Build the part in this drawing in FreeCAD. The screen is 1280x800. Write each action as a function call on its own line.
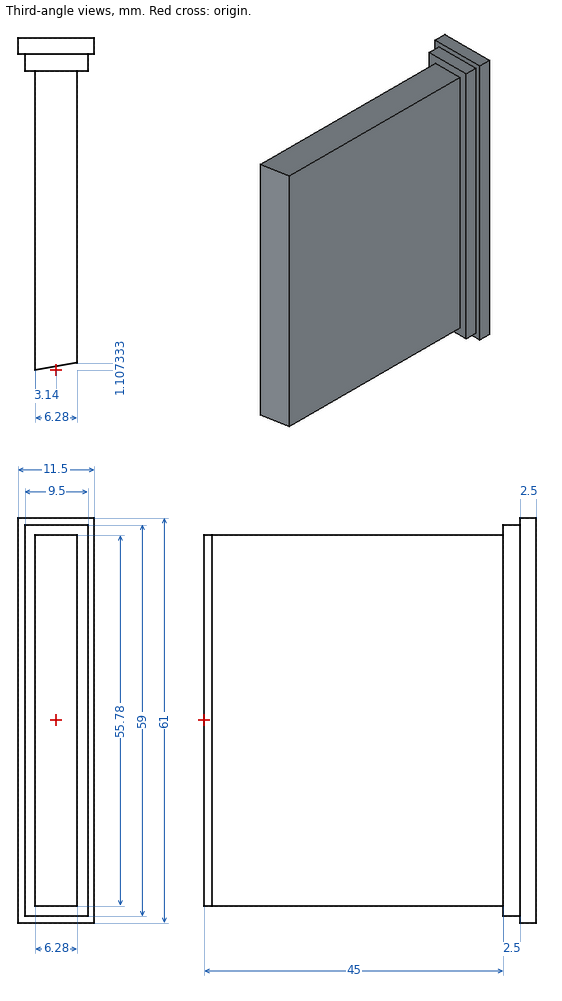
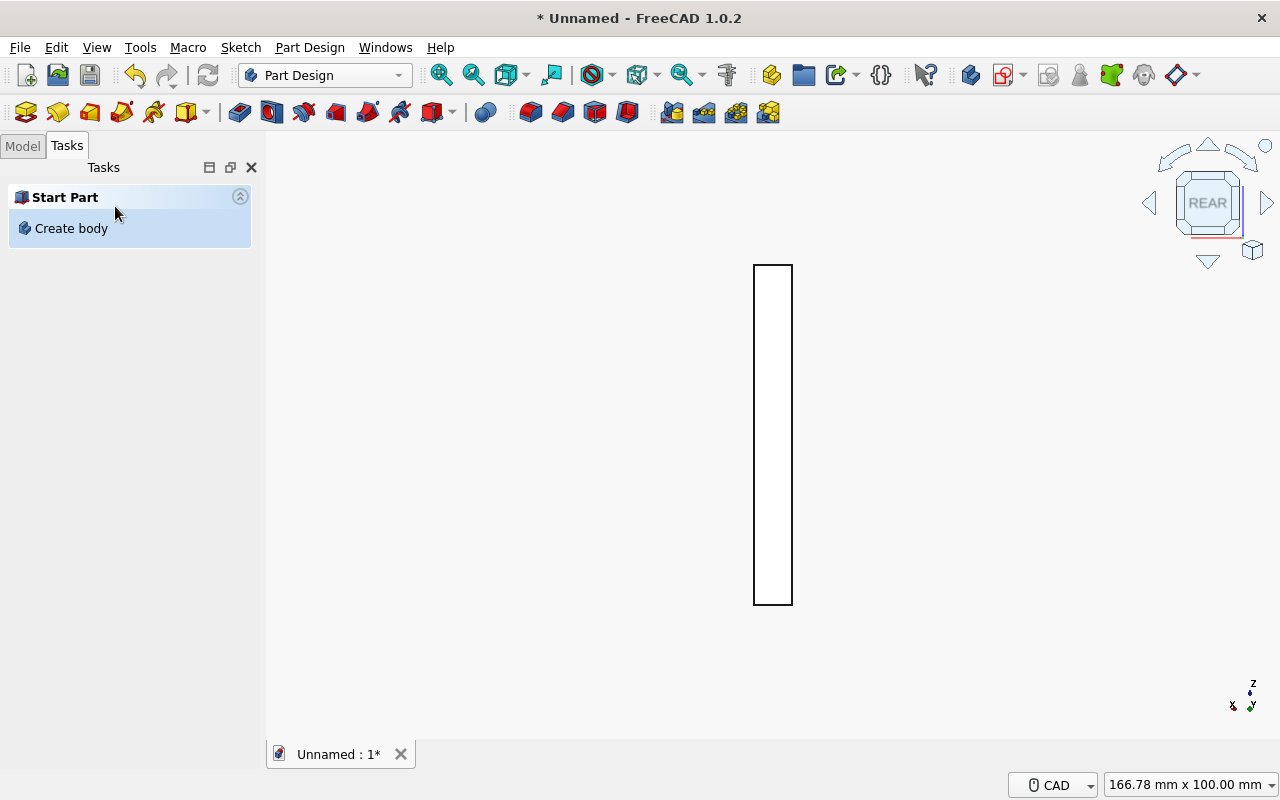
click(773, 289)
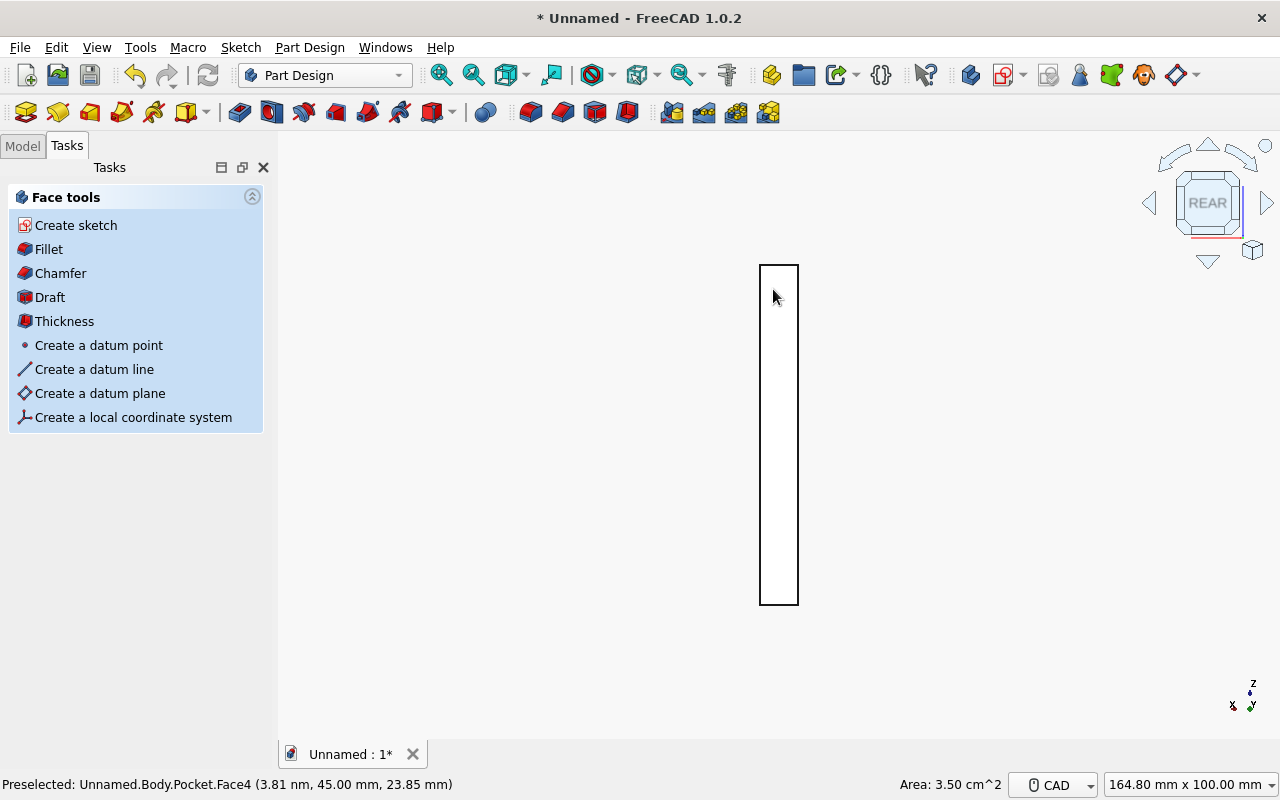
click(1004, 76)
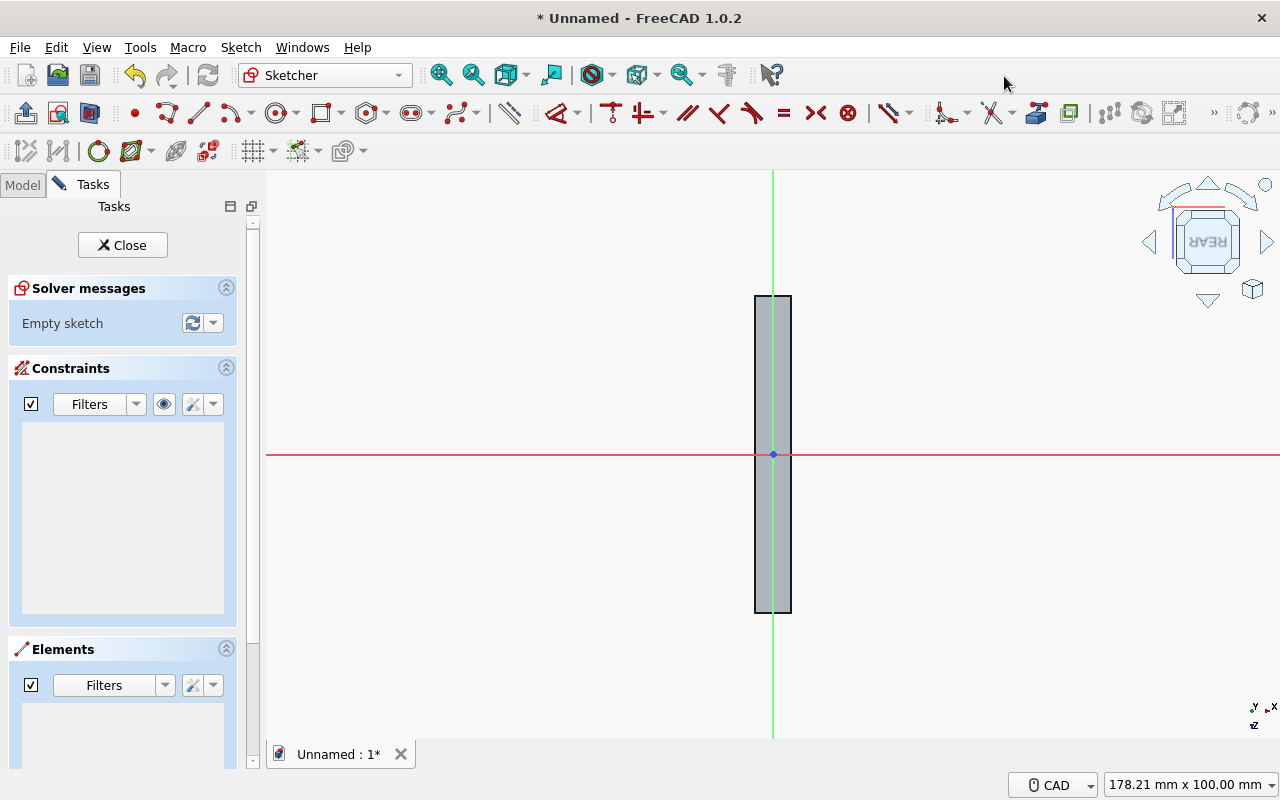
key(g)
key(v)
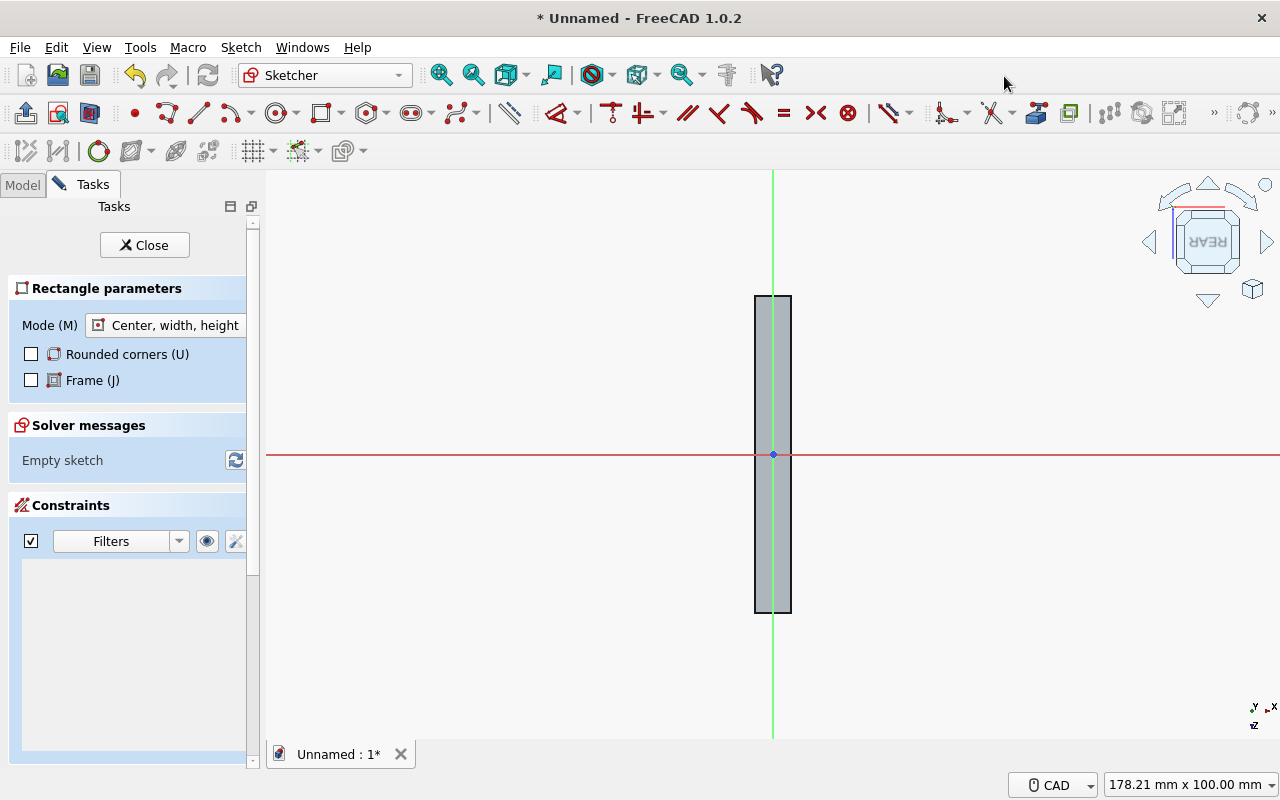
click(773, 455)
move(800, 287)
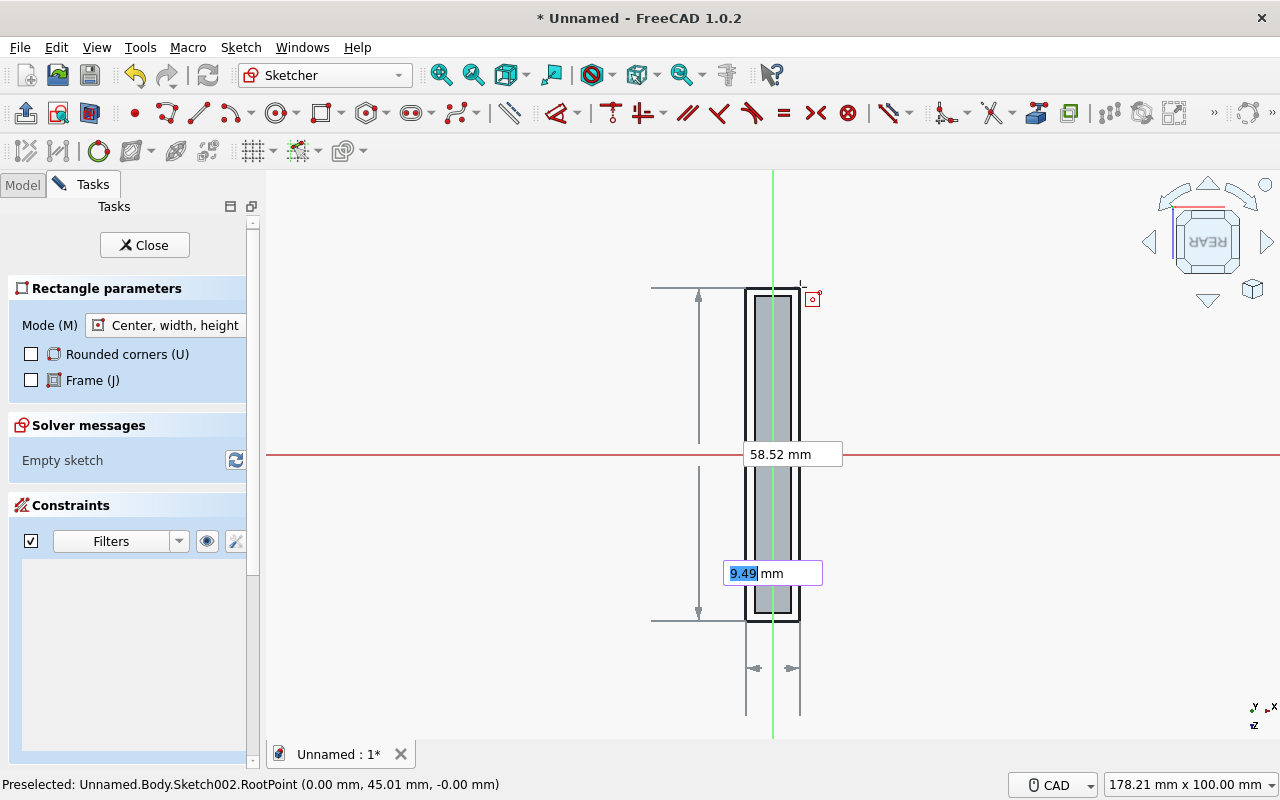
text(9.5)
key(Tab)
text(59)
key(Return)
key(Escape)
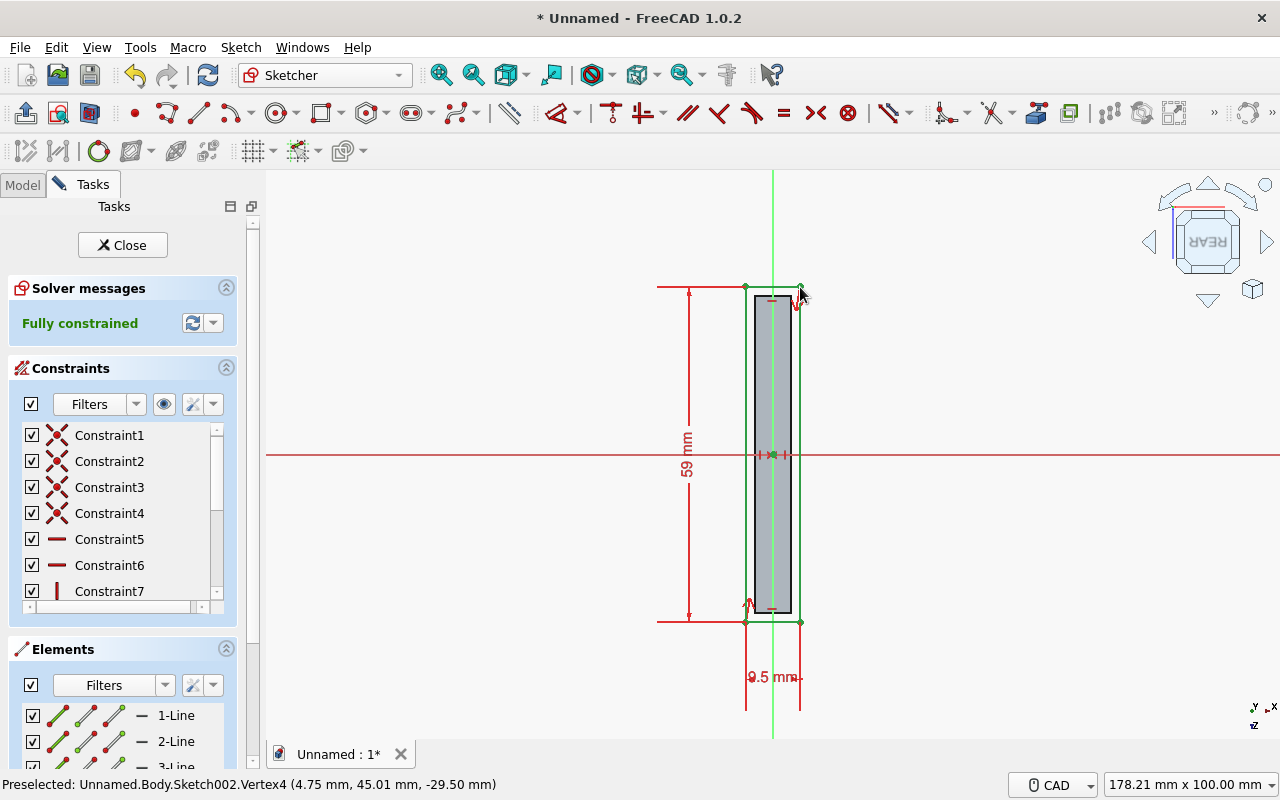
click(123, 245)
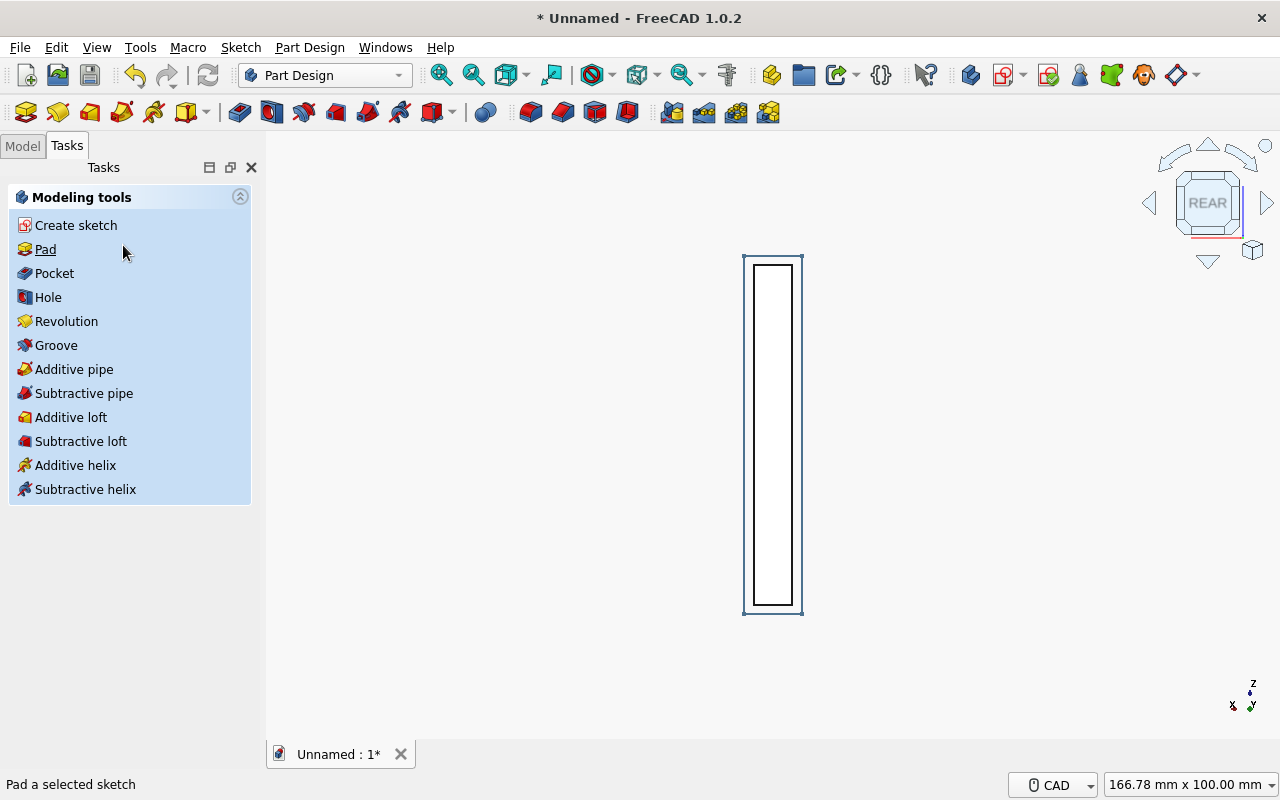
click(26, 112)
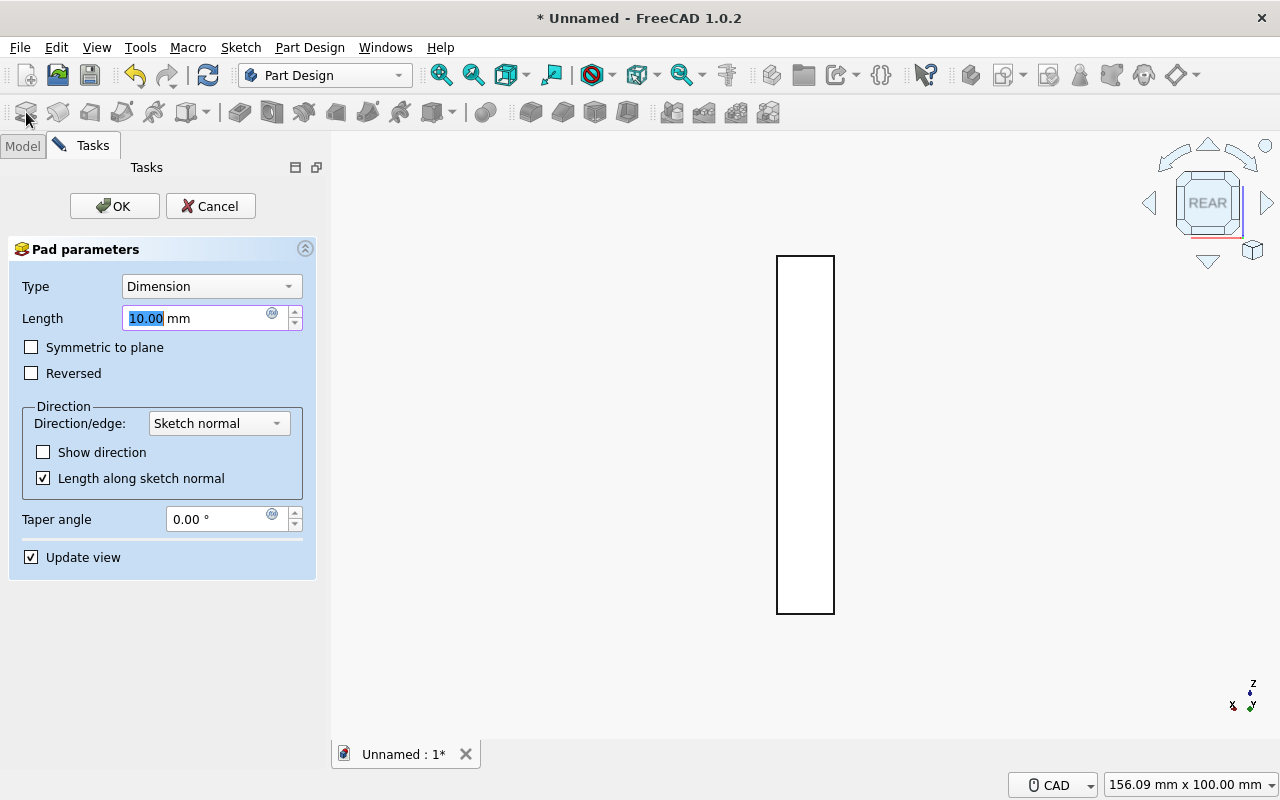
text(2.5)
key(Tab)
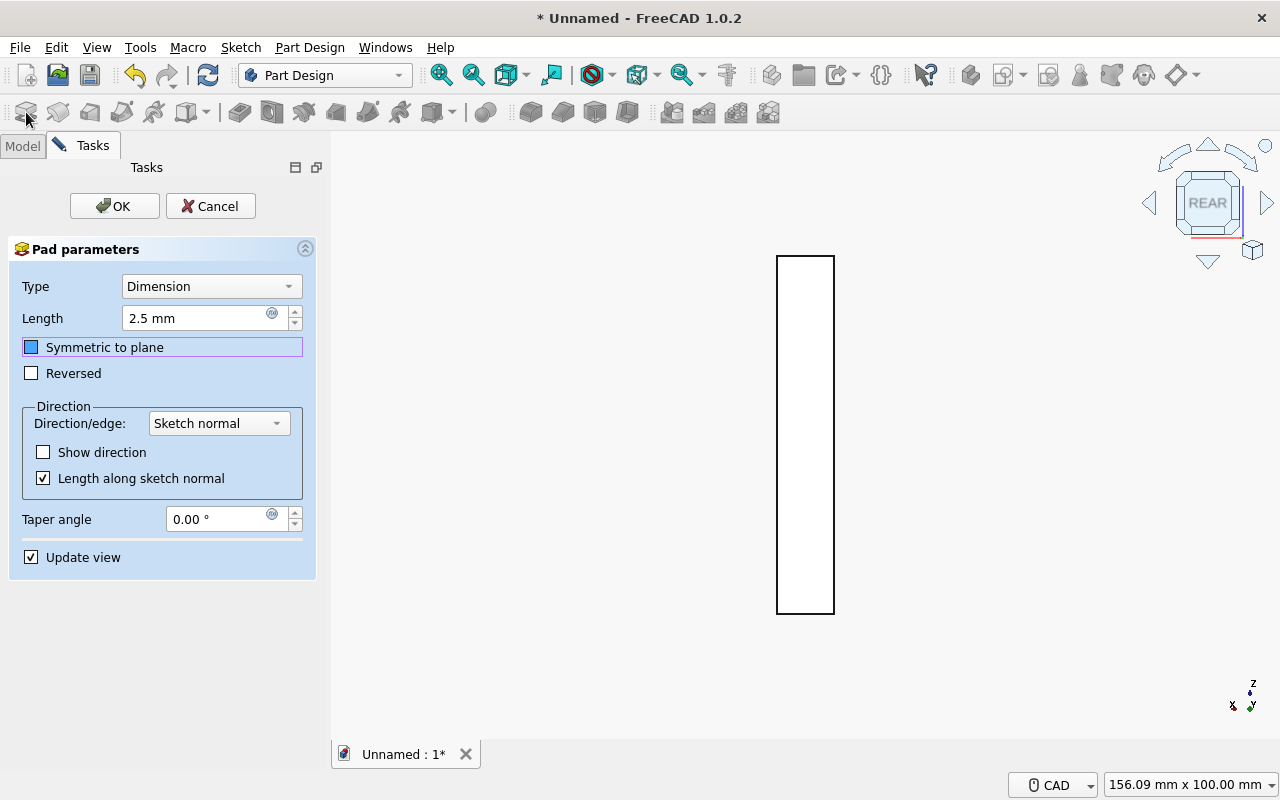
click(115, 206)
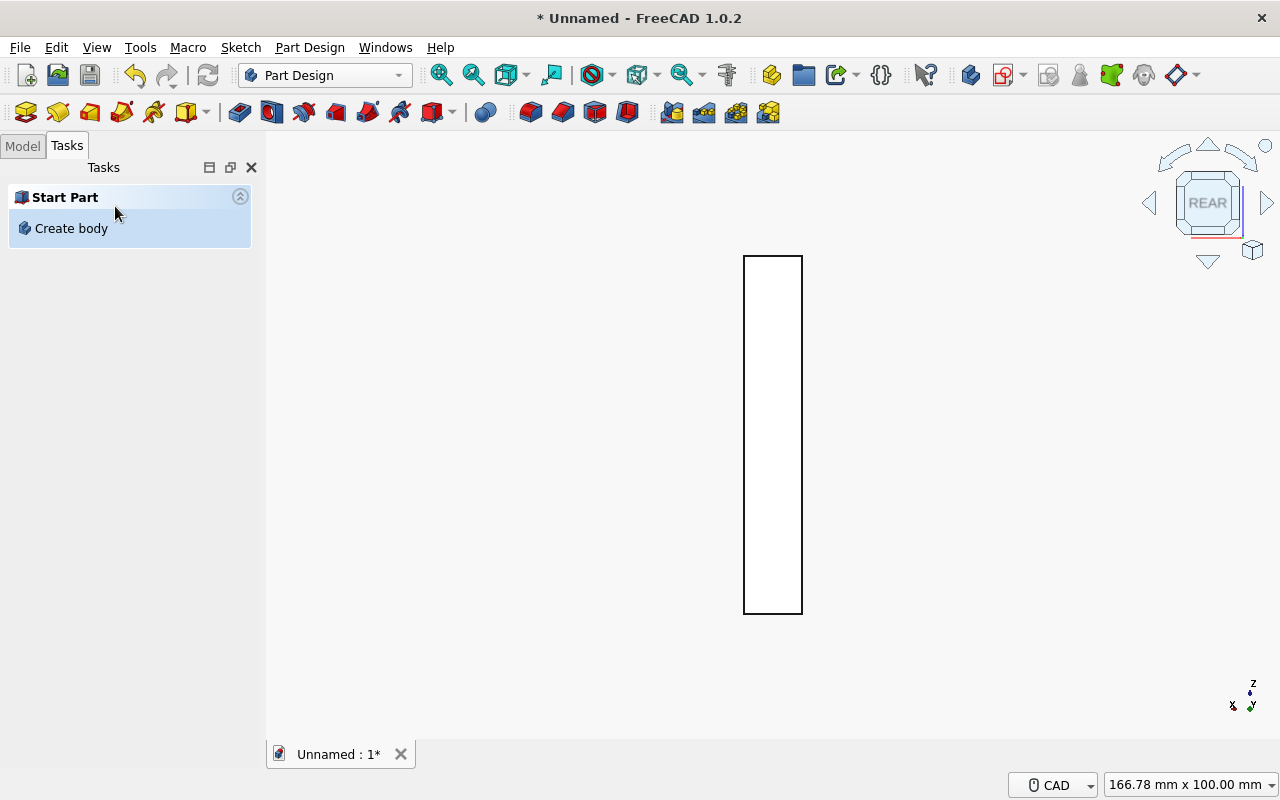
click(773, 536)